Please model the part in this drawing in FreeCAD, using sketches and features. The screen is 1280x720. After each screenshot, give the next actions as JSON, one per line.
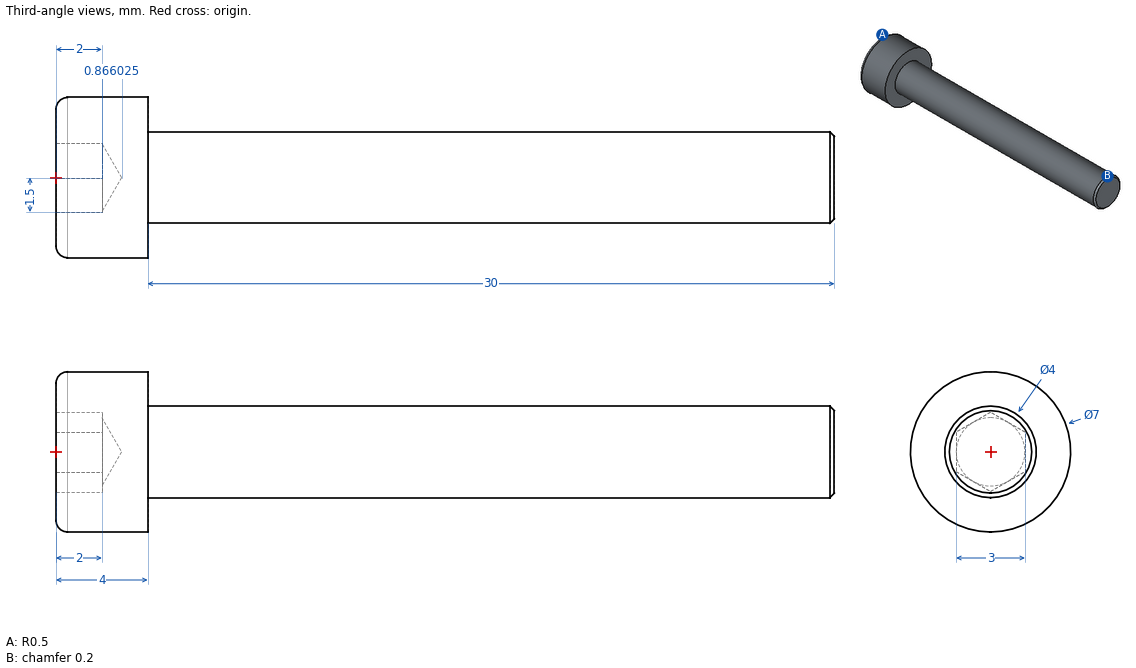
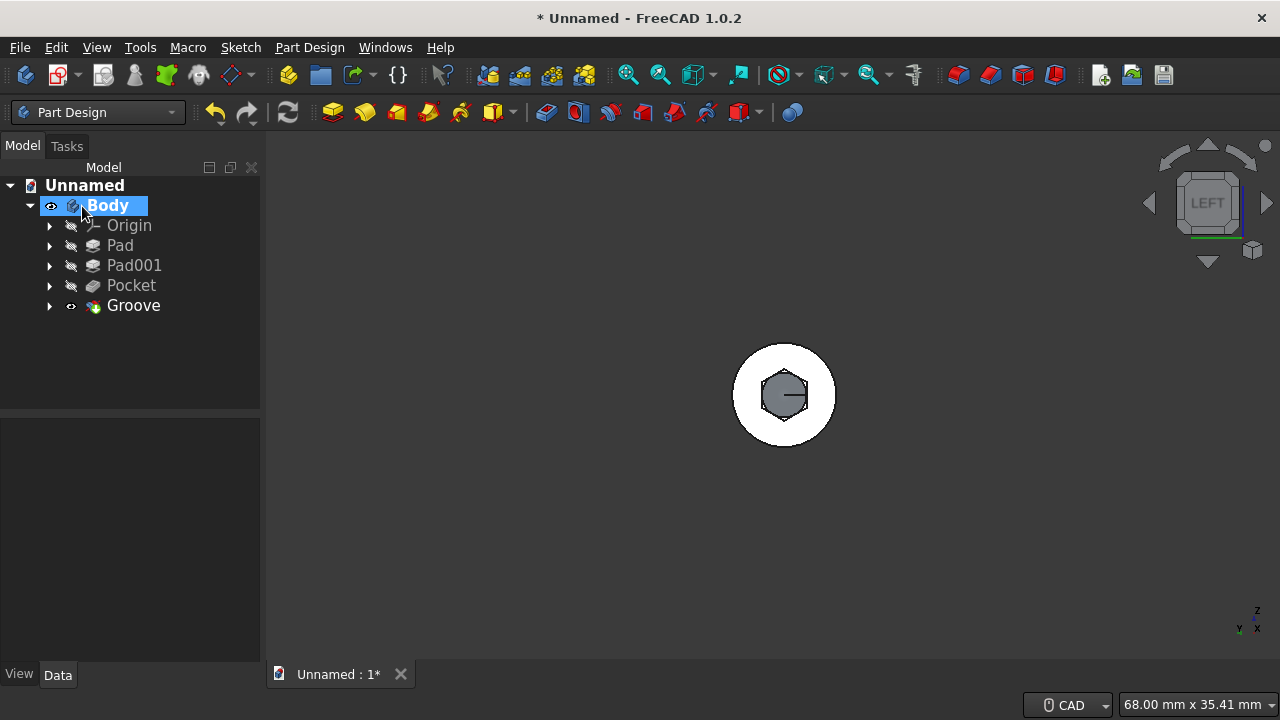
{"action": "left_click", "coordinate": [630, 76]}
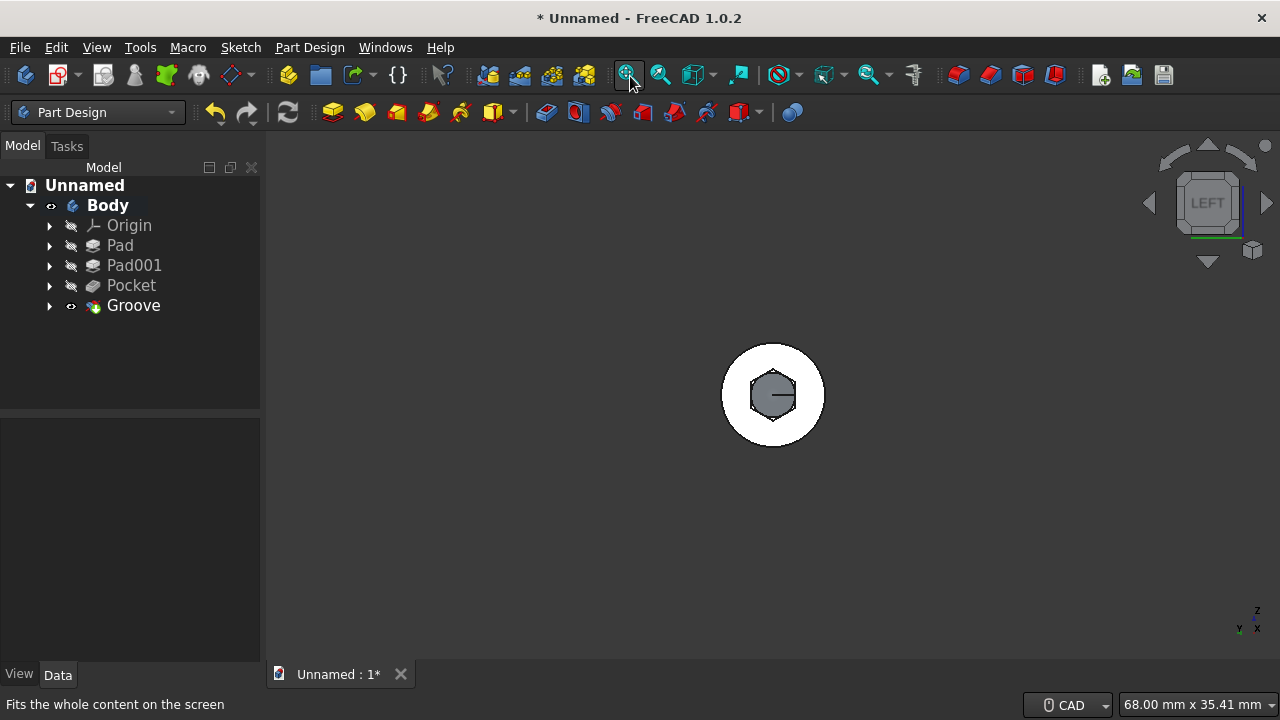
{"action": "left_click", "coordinate": [815, 363]}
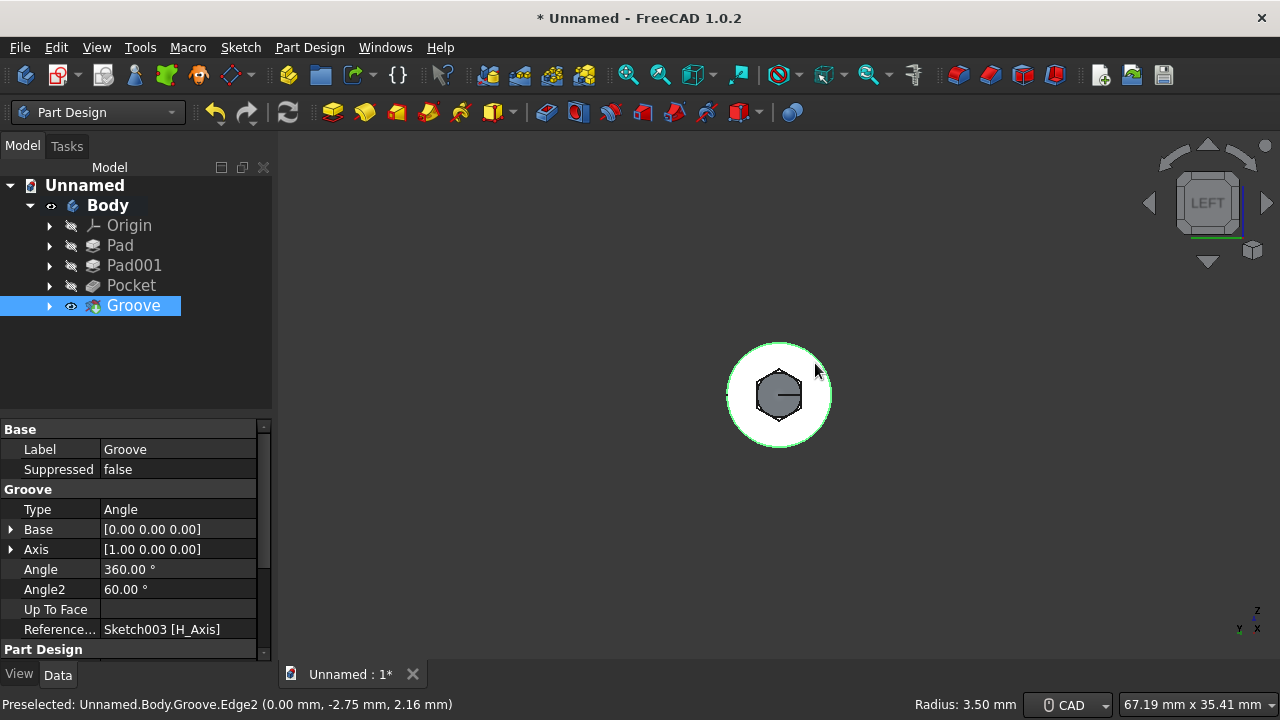
{"action": "left_click", "coordinate": [960, 76]}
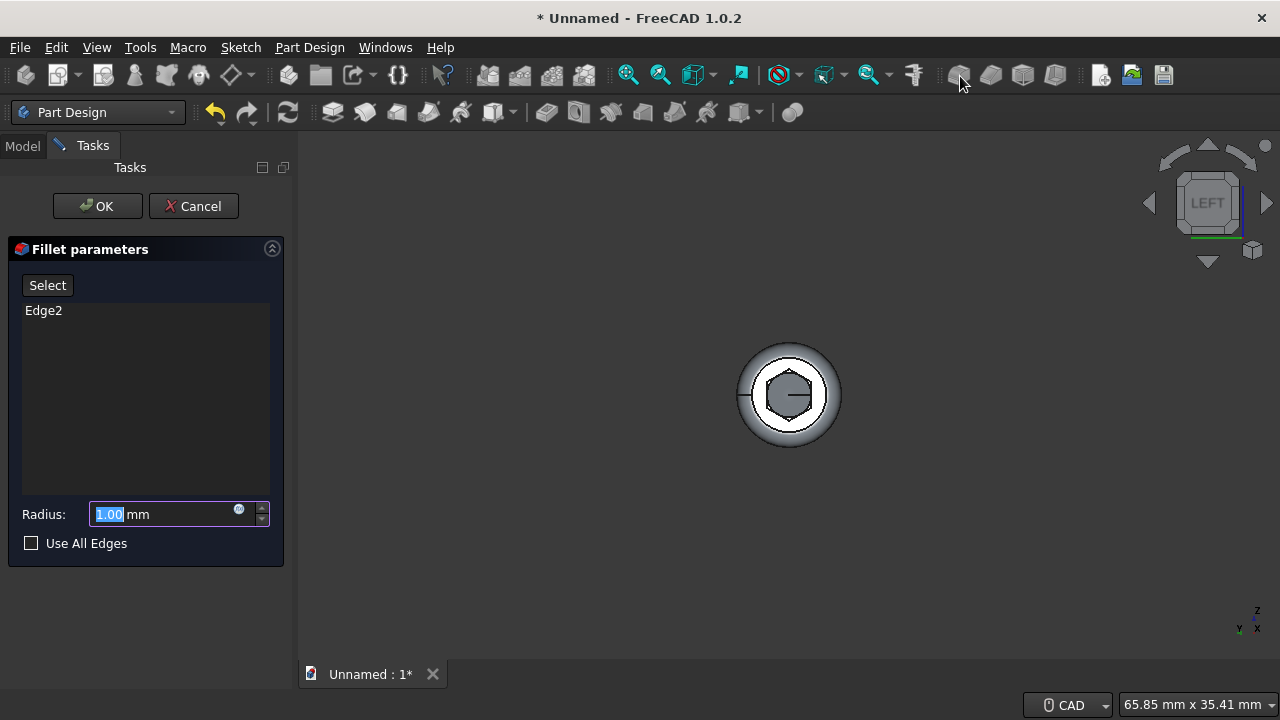
{"action": "type", "text": "0.5"}
{"action": "key", "text": "Tab"}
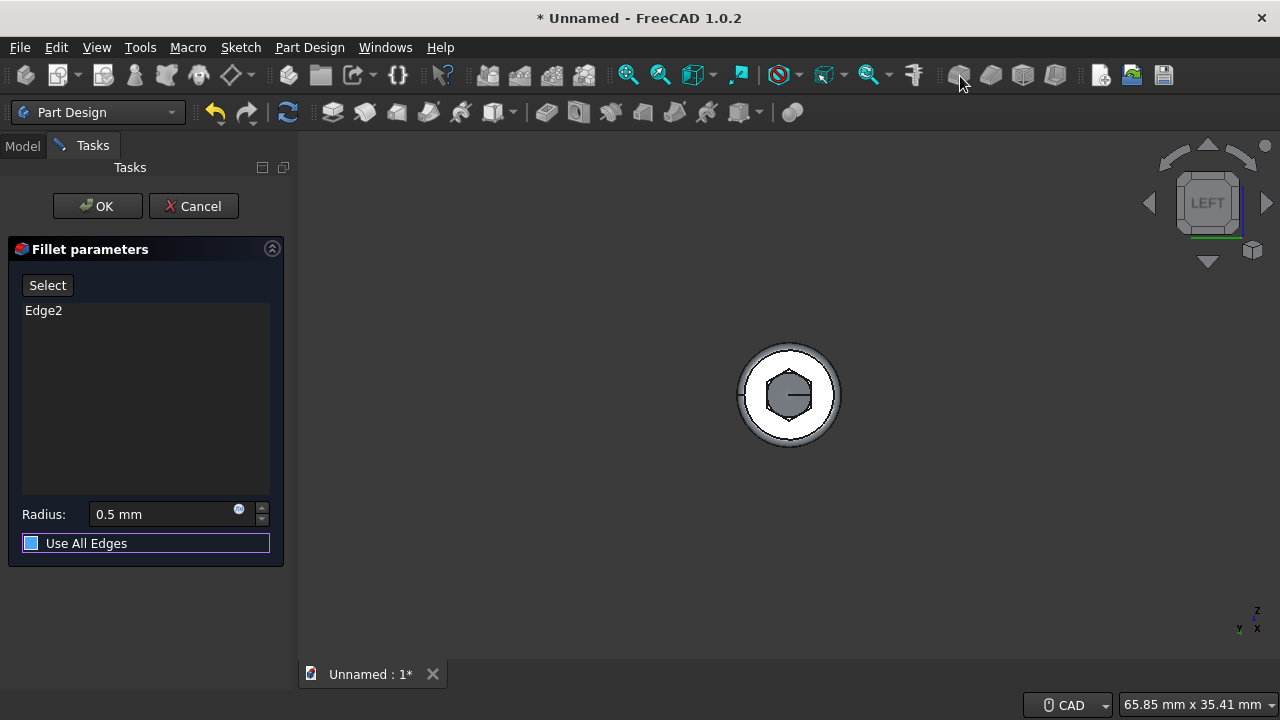
{"action": "left_click", "coordinate": [98, 206]}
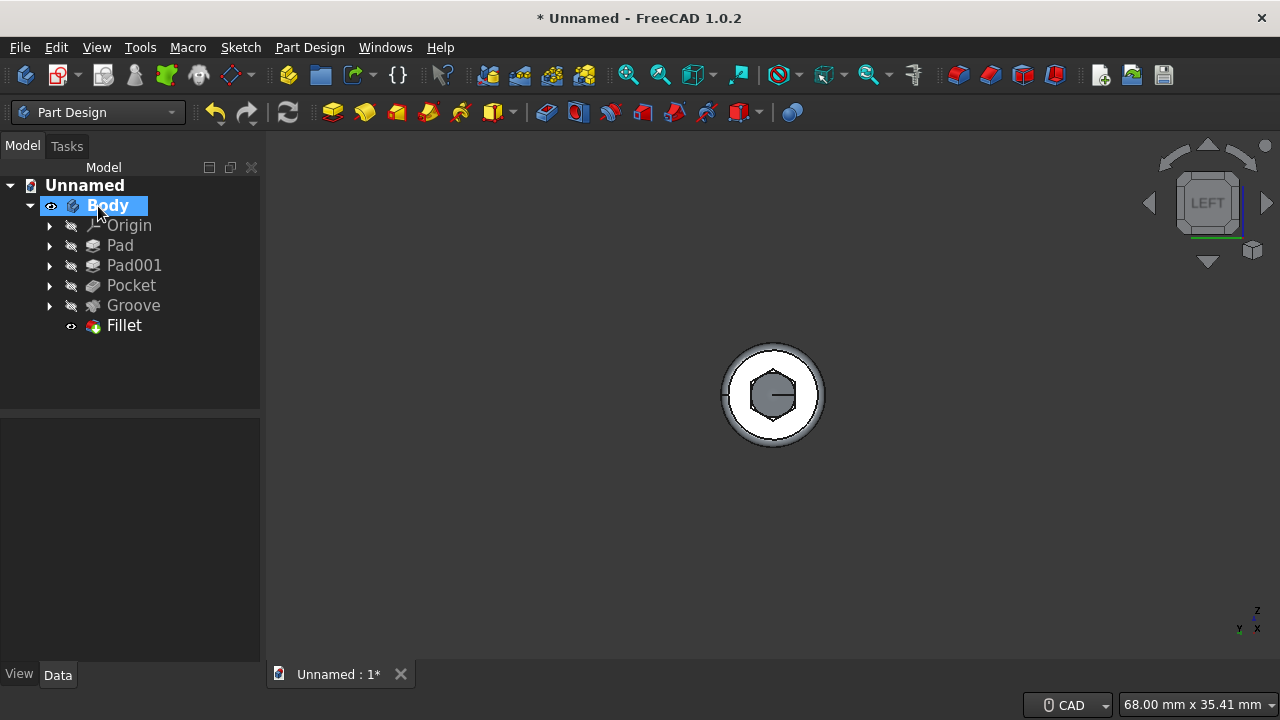
{"action": "left_click", "coordinate": [630, 76]}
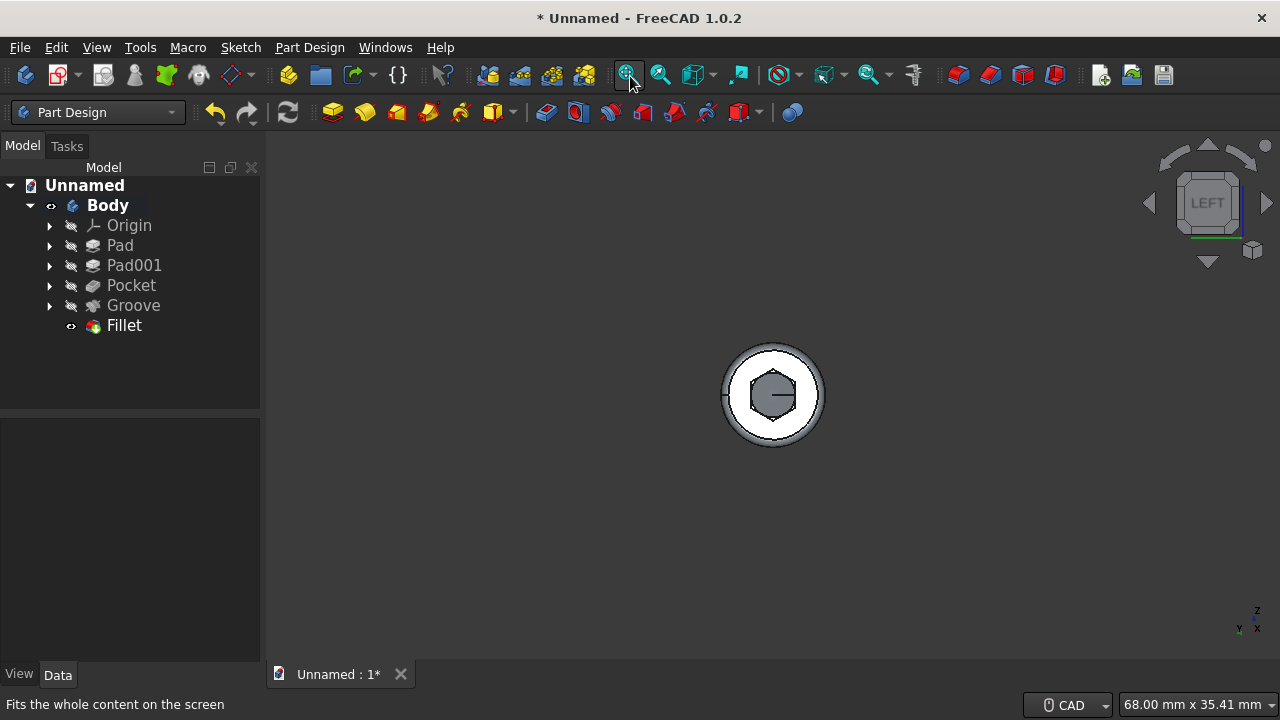
{"action": "key", "text": "0"}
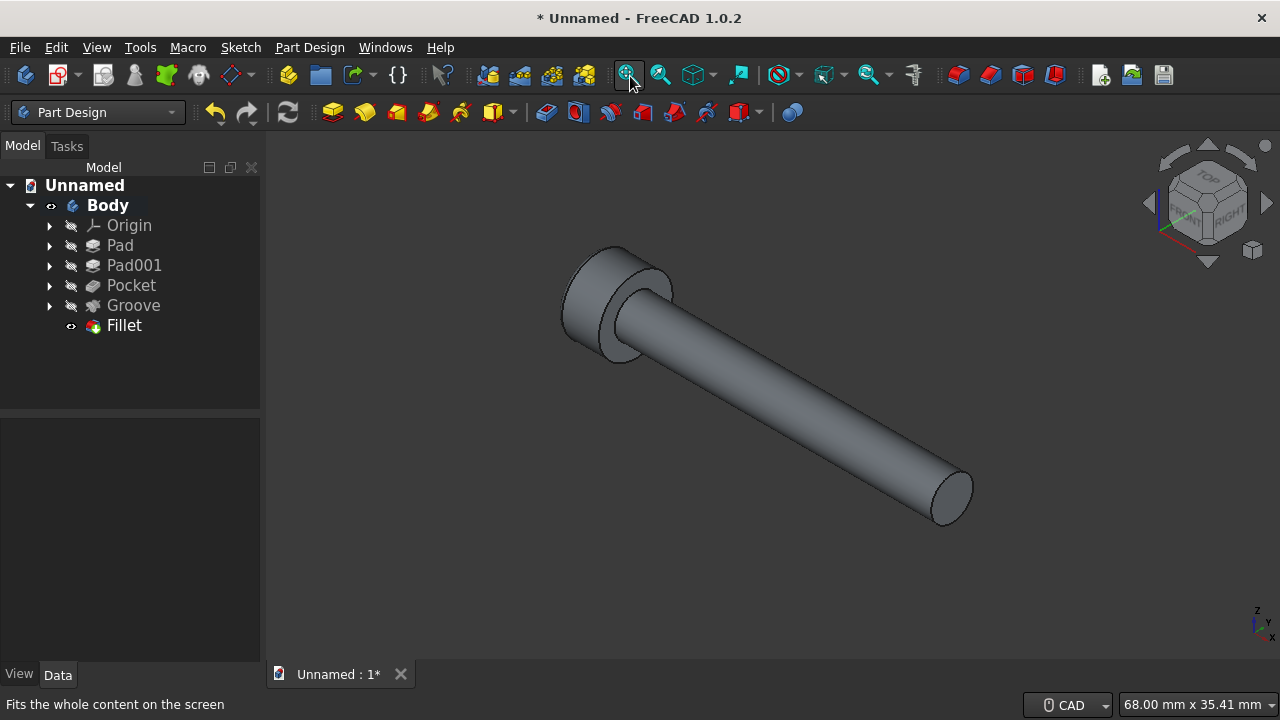
{"action": "left_click", "coordinate": [931, 510]}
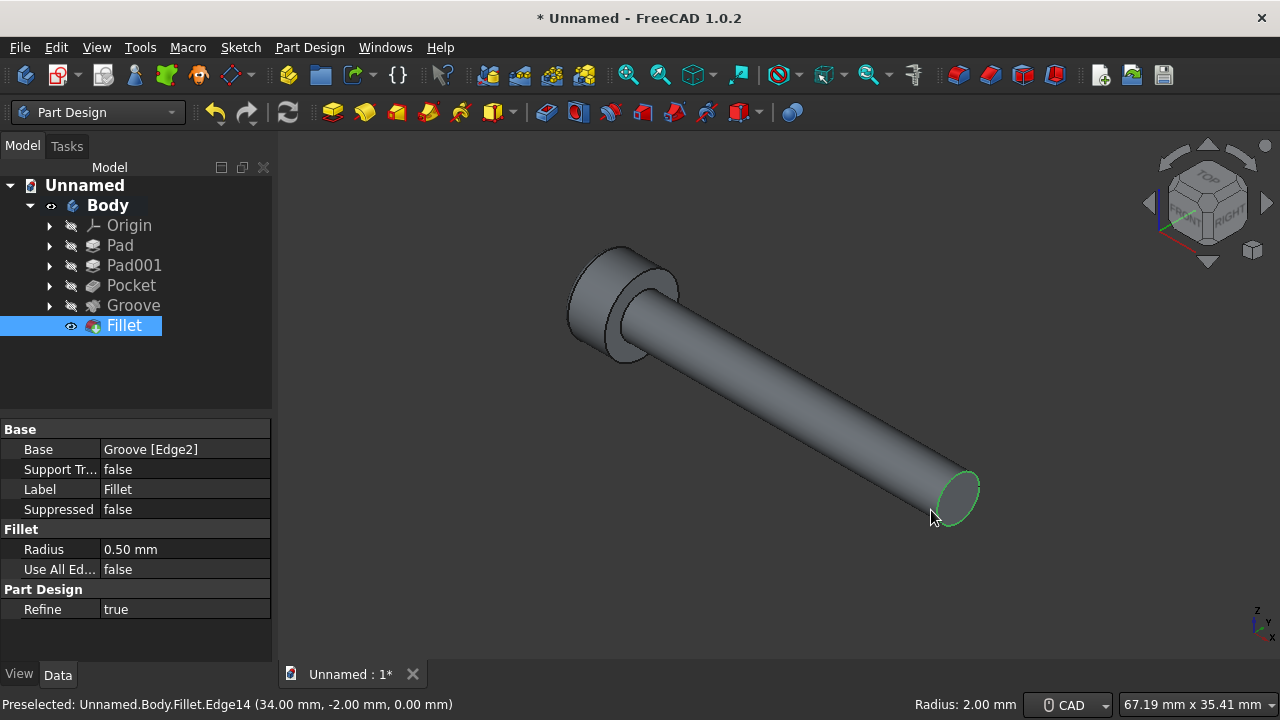
{"action": "left_click", "coordinate": [992, 76]}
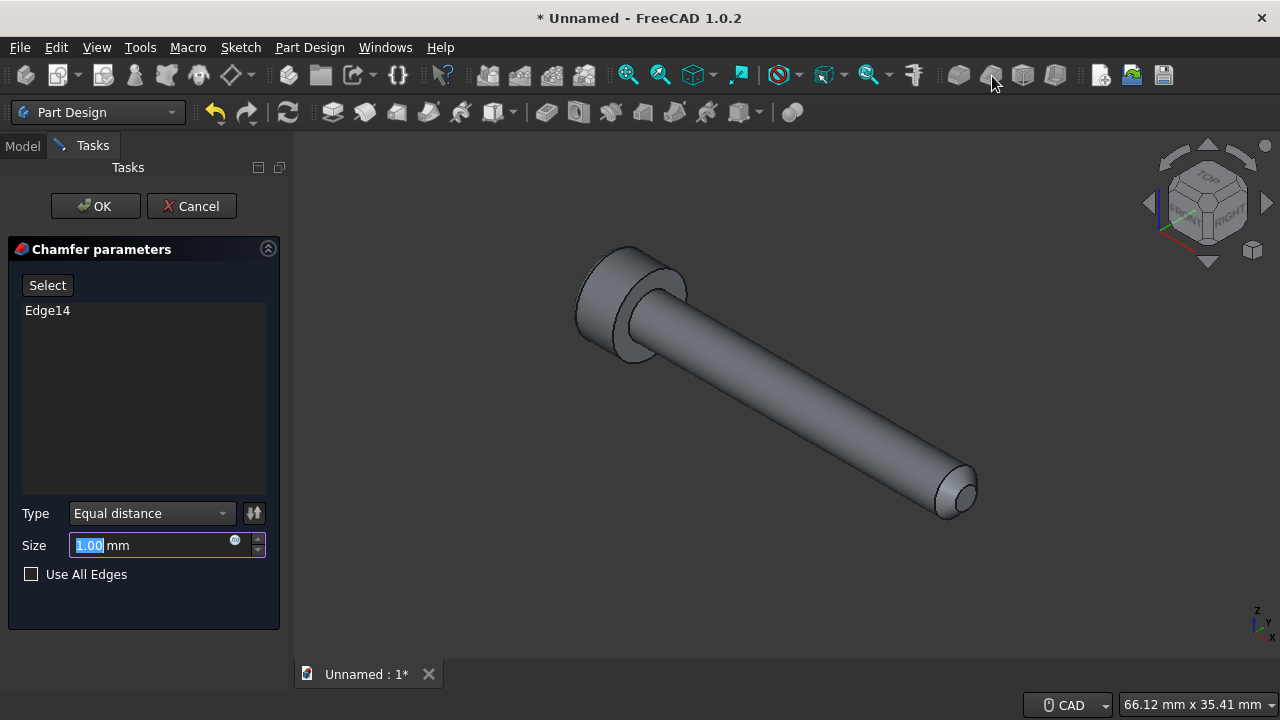
{"action": "type", "text": "0.2"}
{"action": "key", "text": "Tab"}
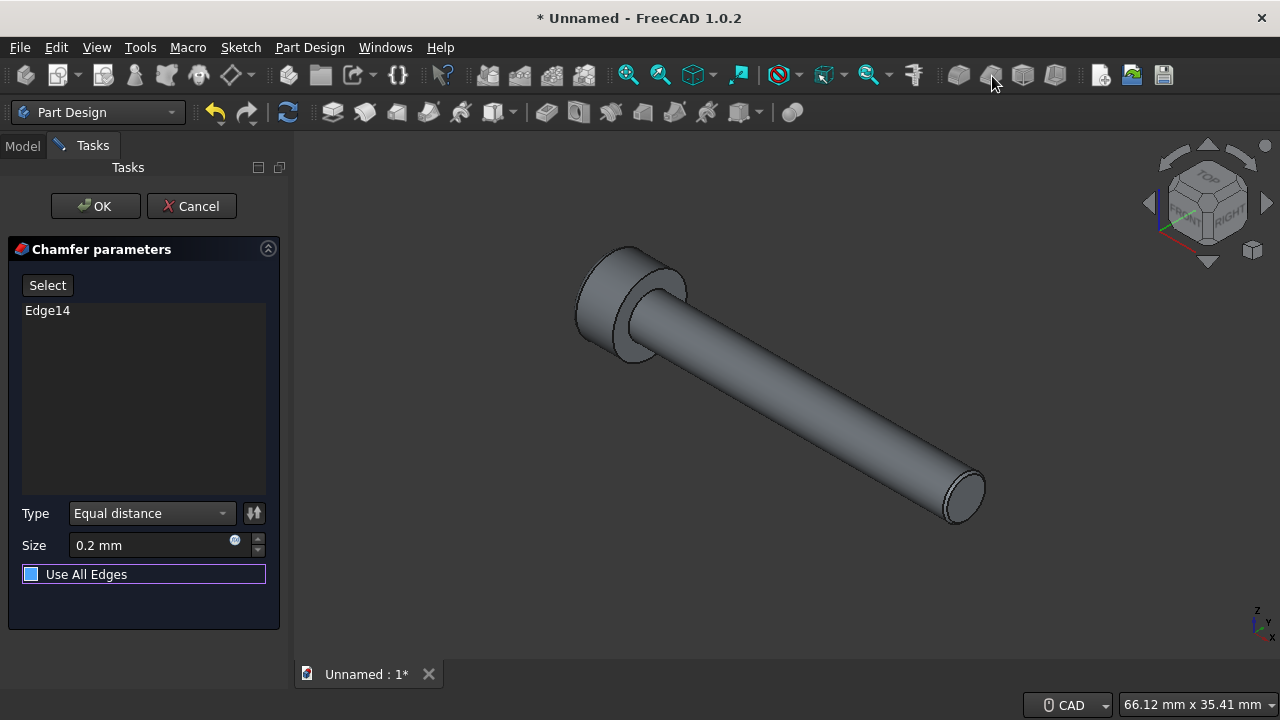
{"action": "left_click", "coordinate": [96, 206]}